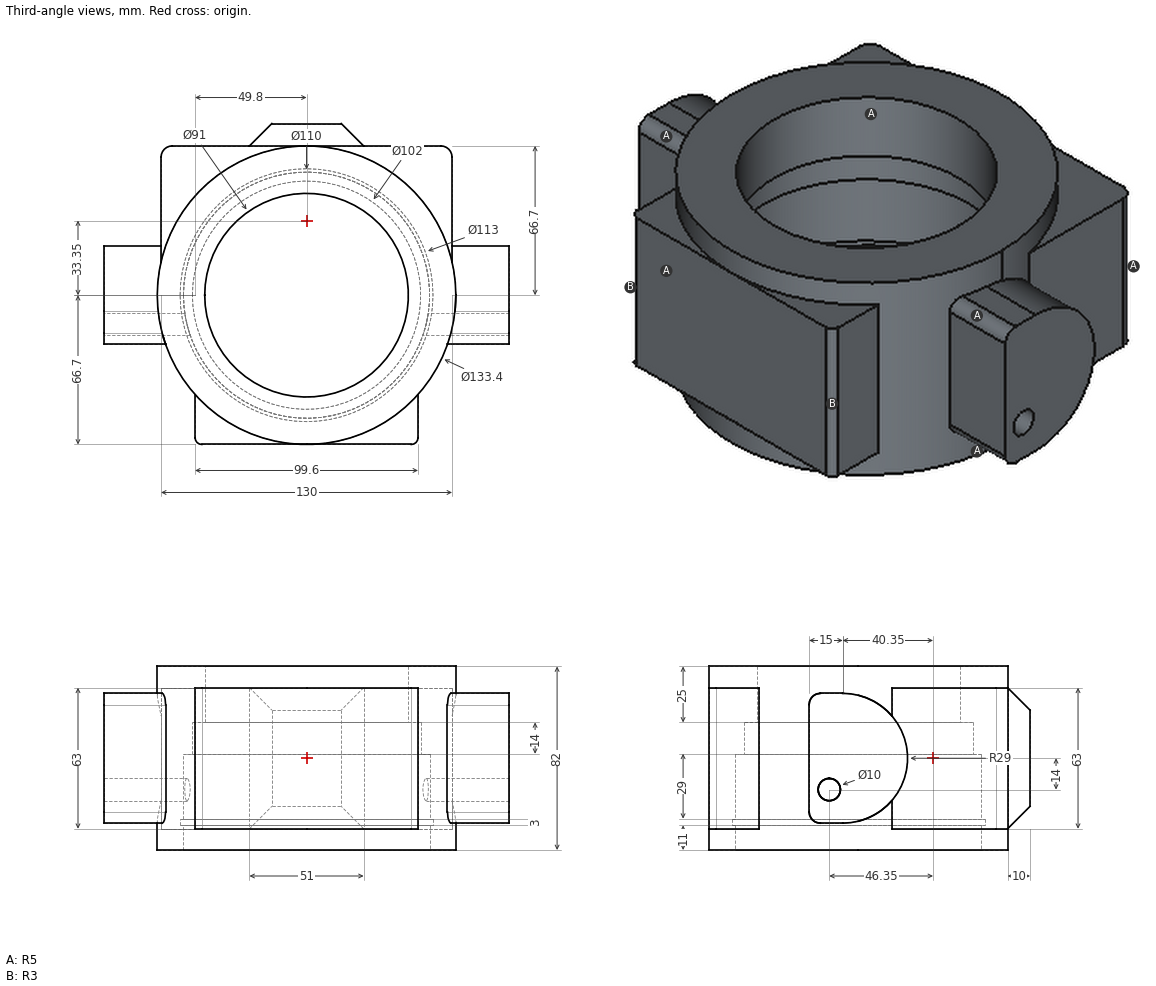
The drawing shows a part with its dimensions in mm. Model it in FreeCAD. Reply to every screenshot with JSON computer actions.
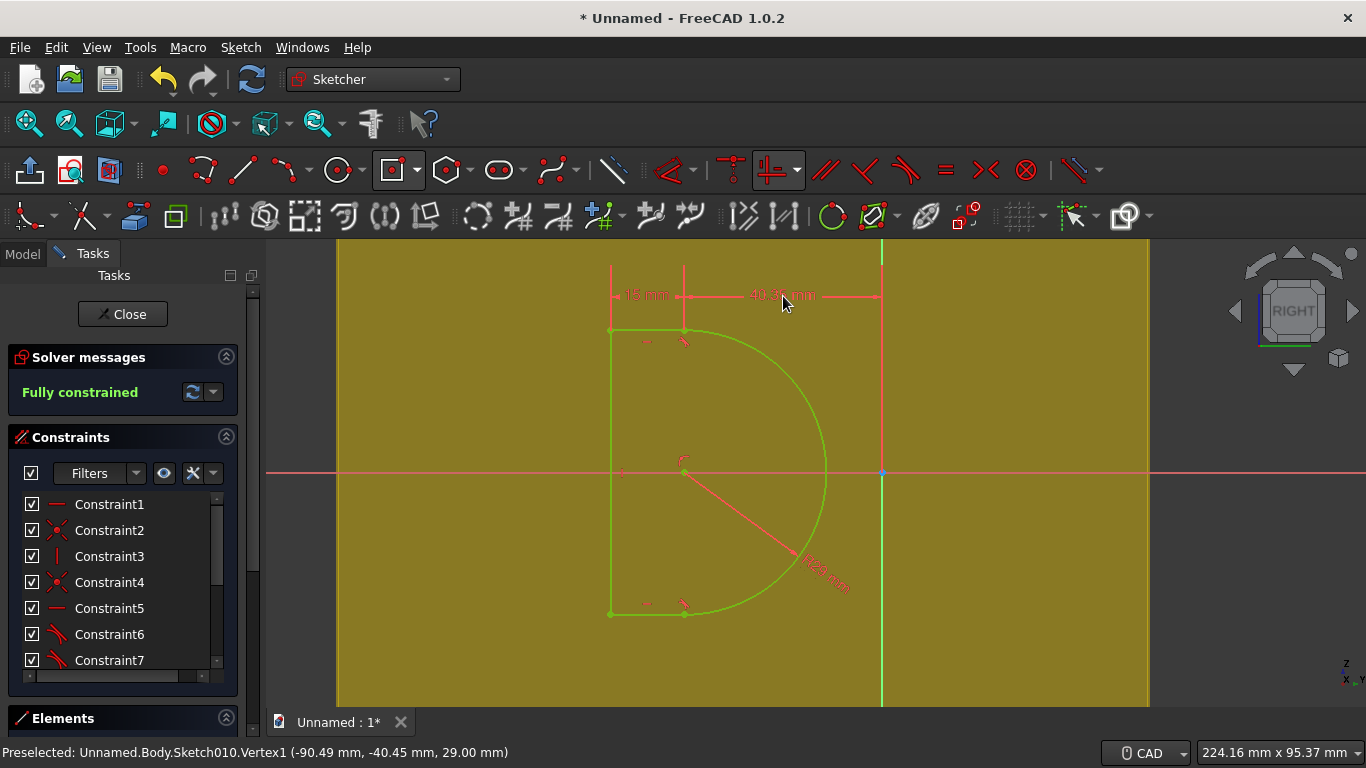
{"action": "left_click", "coordinate": [123, 314]}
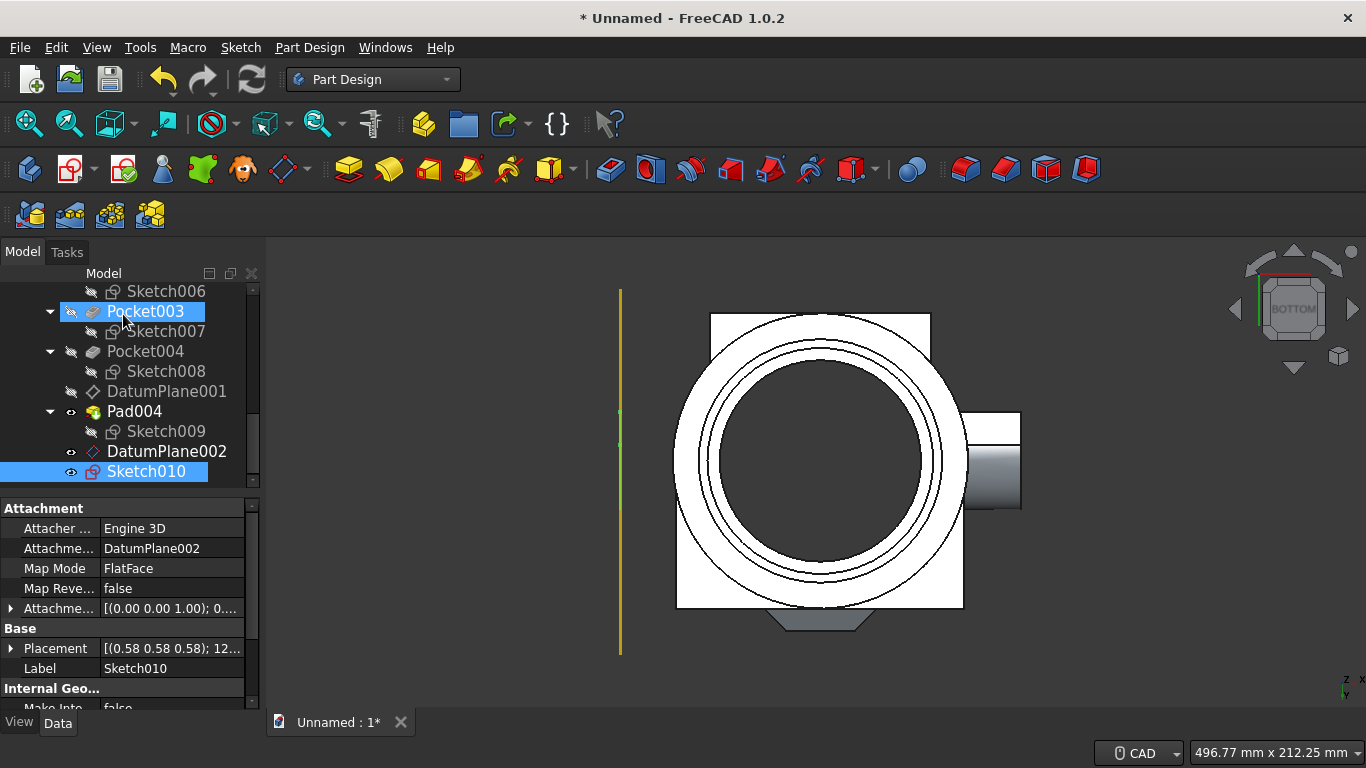
{"action": "left_click", "coordinate": [350, 170]}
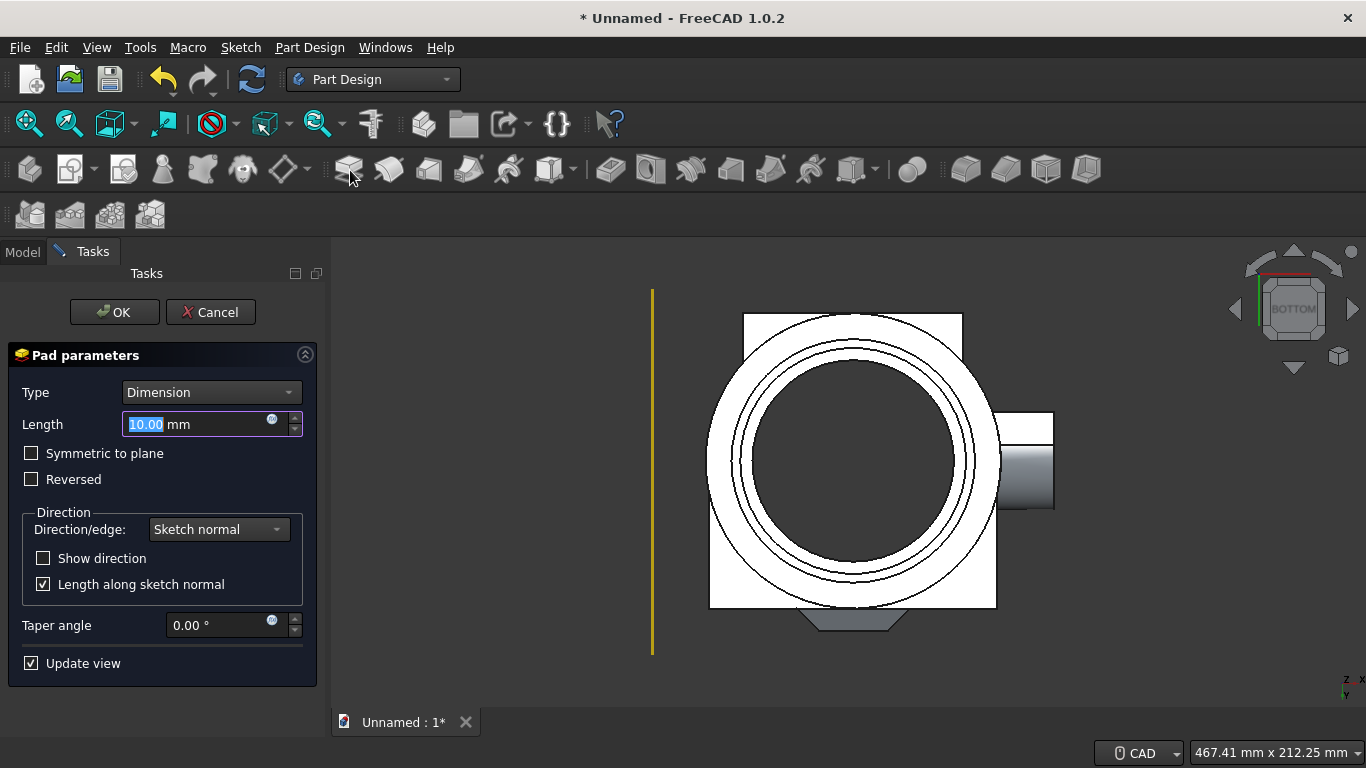
{"action": "left_click", "coordinate": [212, 392]}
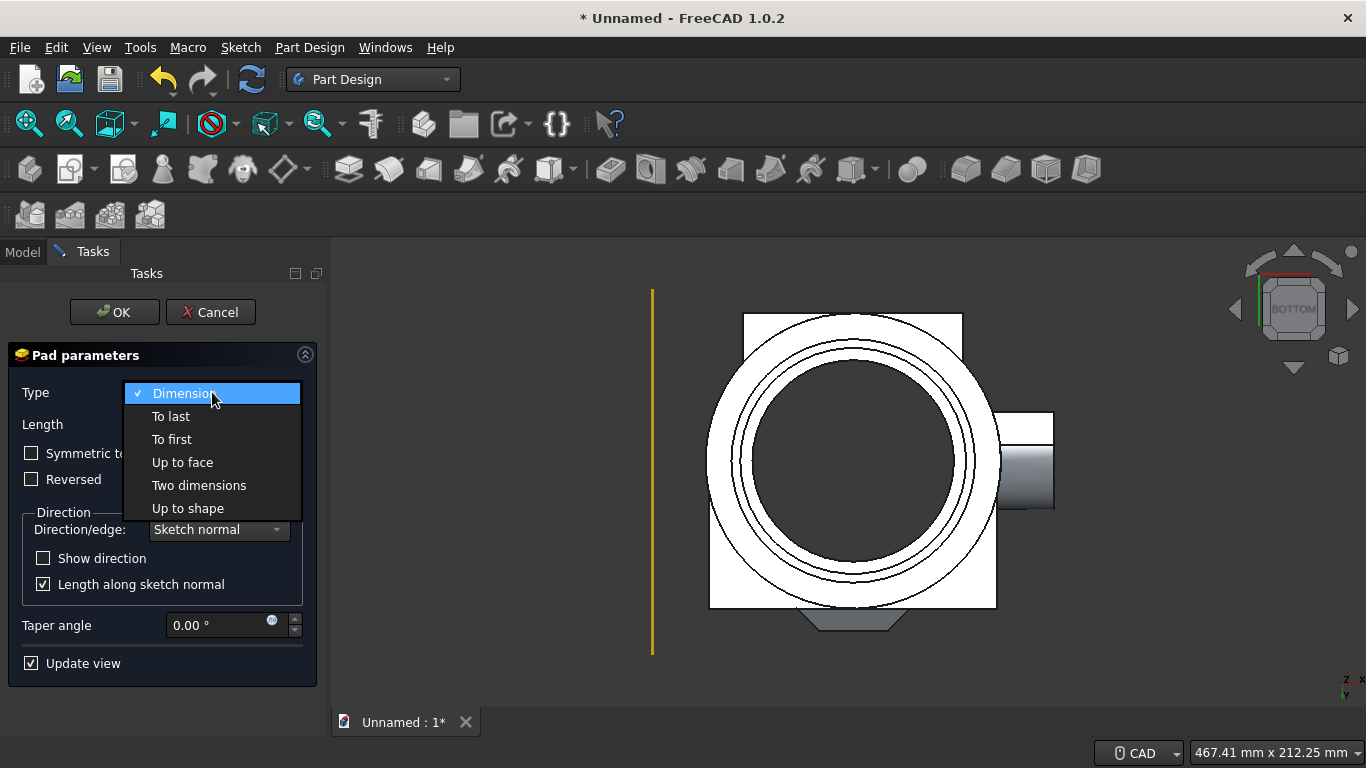
{"action": "left_click", "coordinate": [212, 440]}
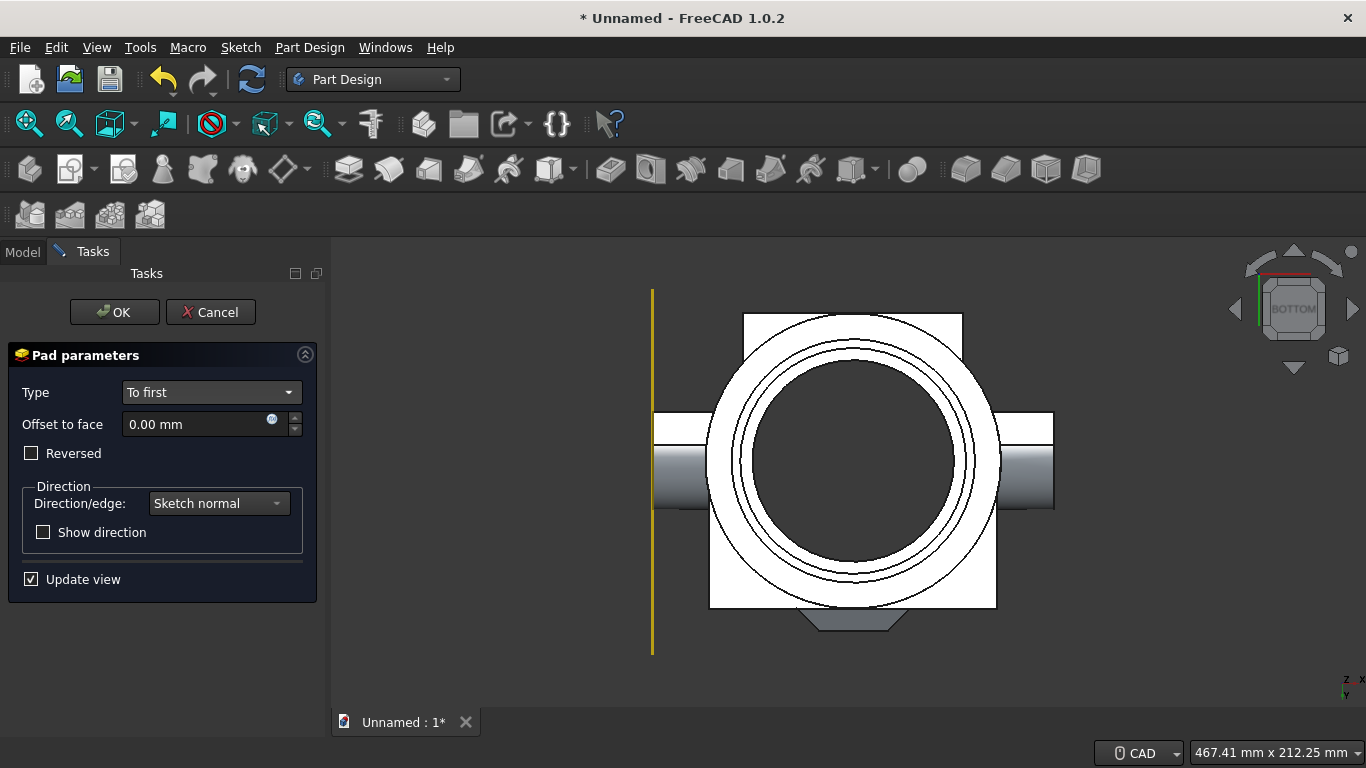
{"action": "left_click", "coordinate": [115, 312]}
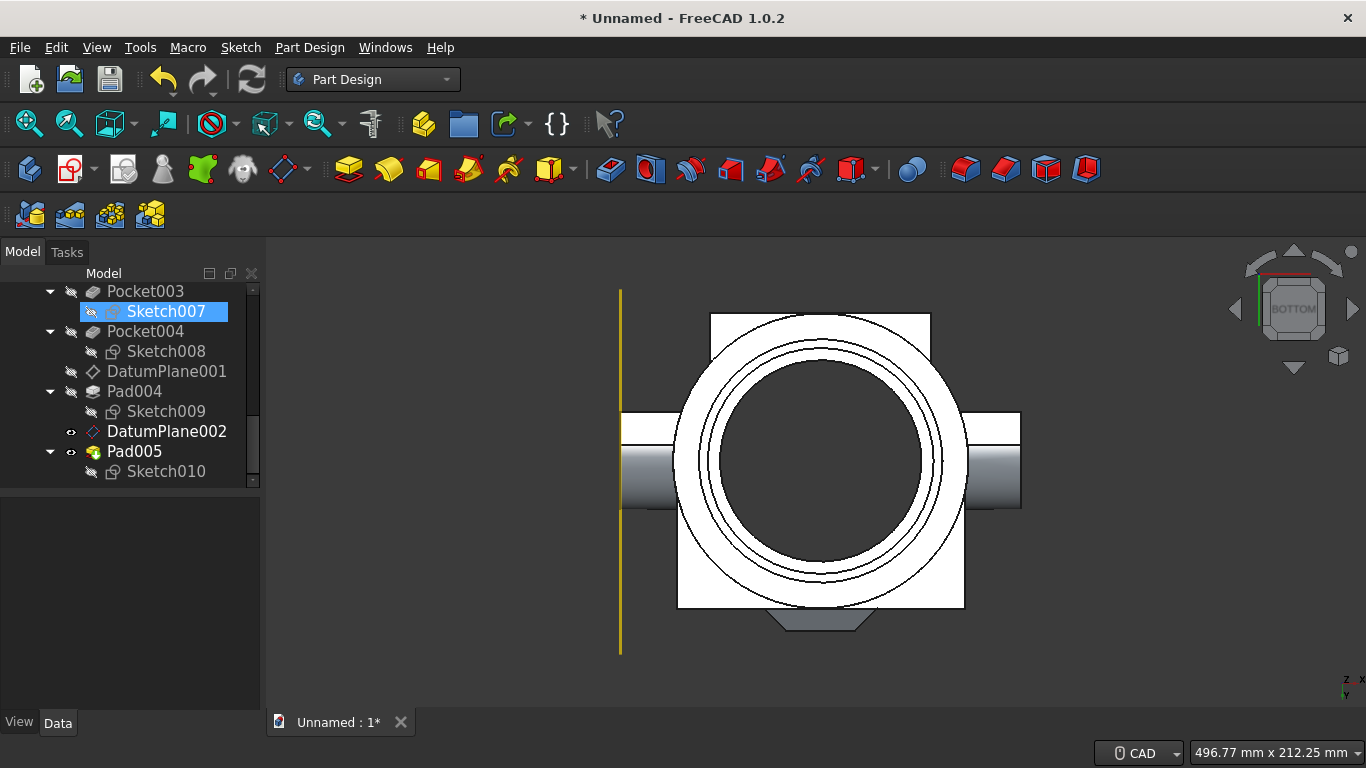
{"action": "left_click", "coordinate": [116, 432]}
{"action": "key", "text": "space"}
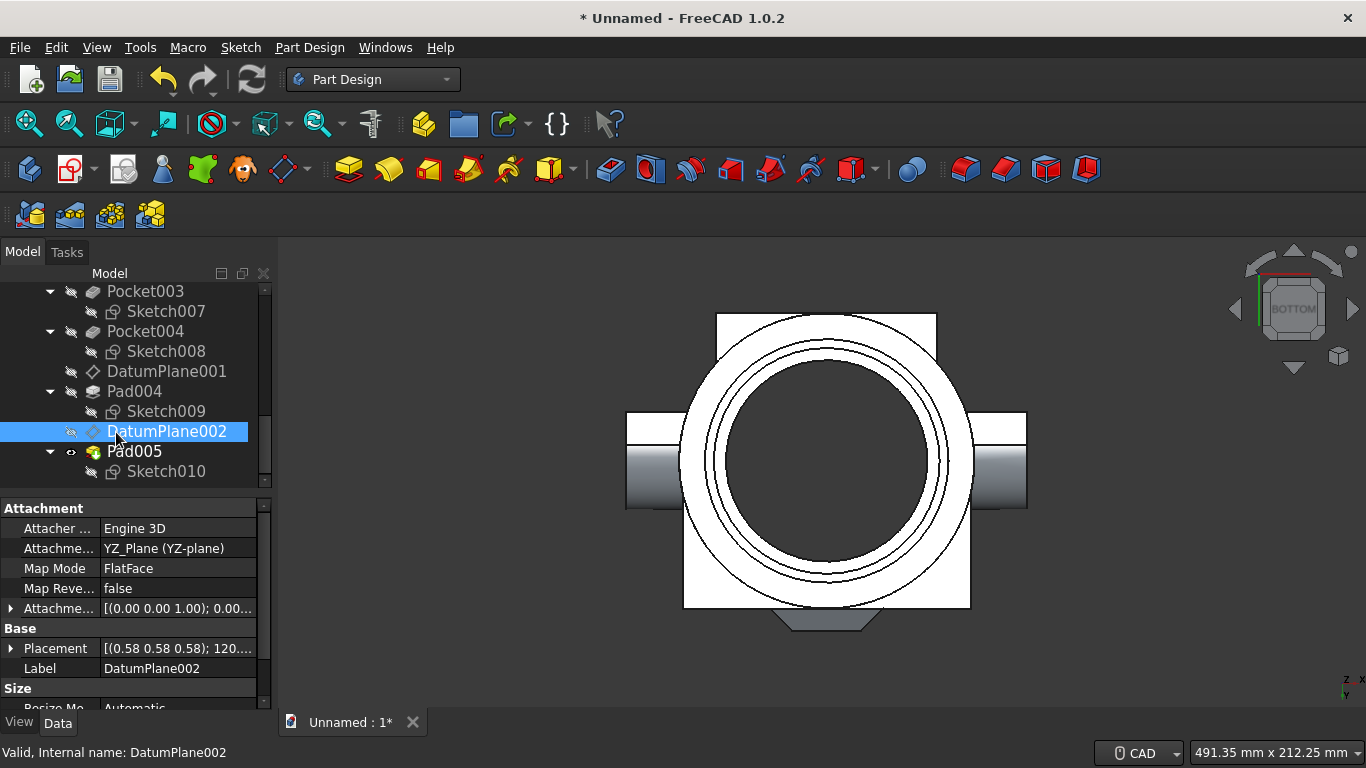
{"action": "key", "text": "6"}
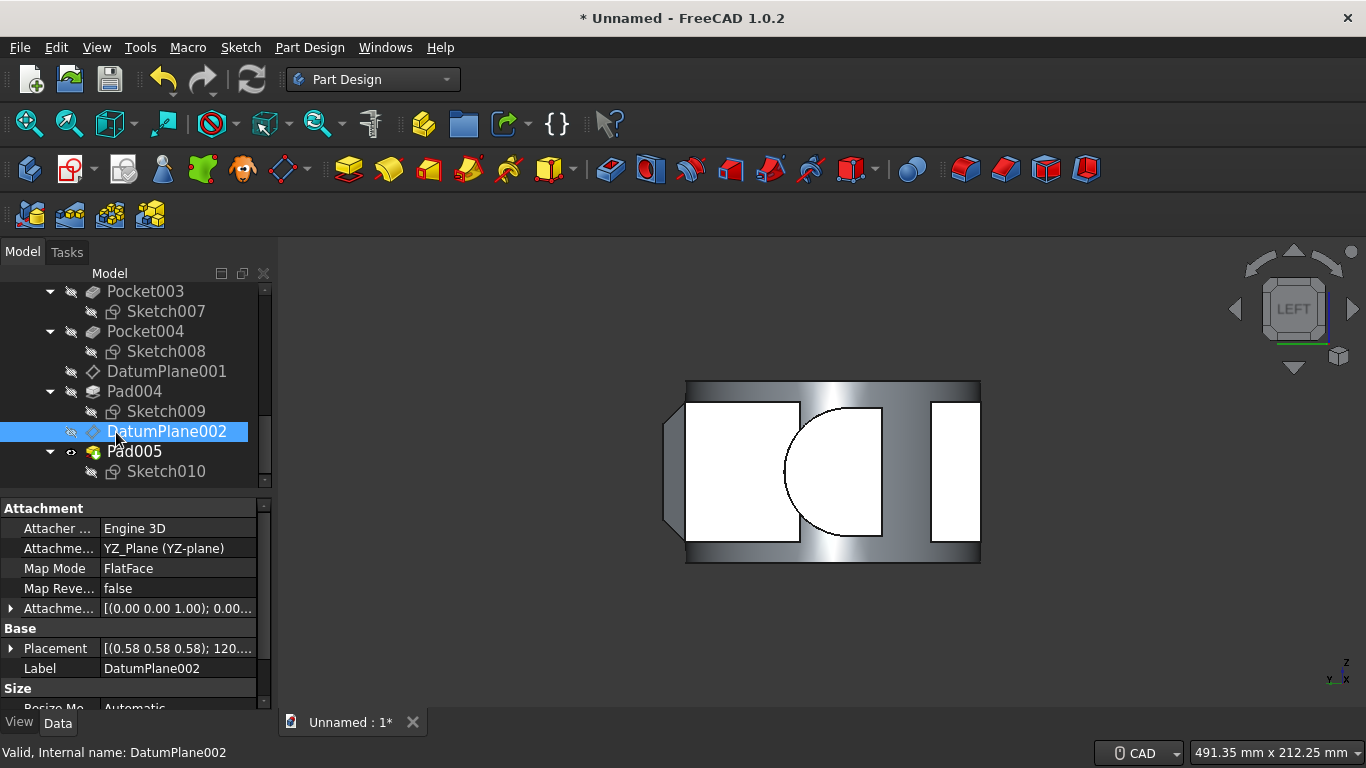
{"action": "left_click", "coordinate": [30, 124]}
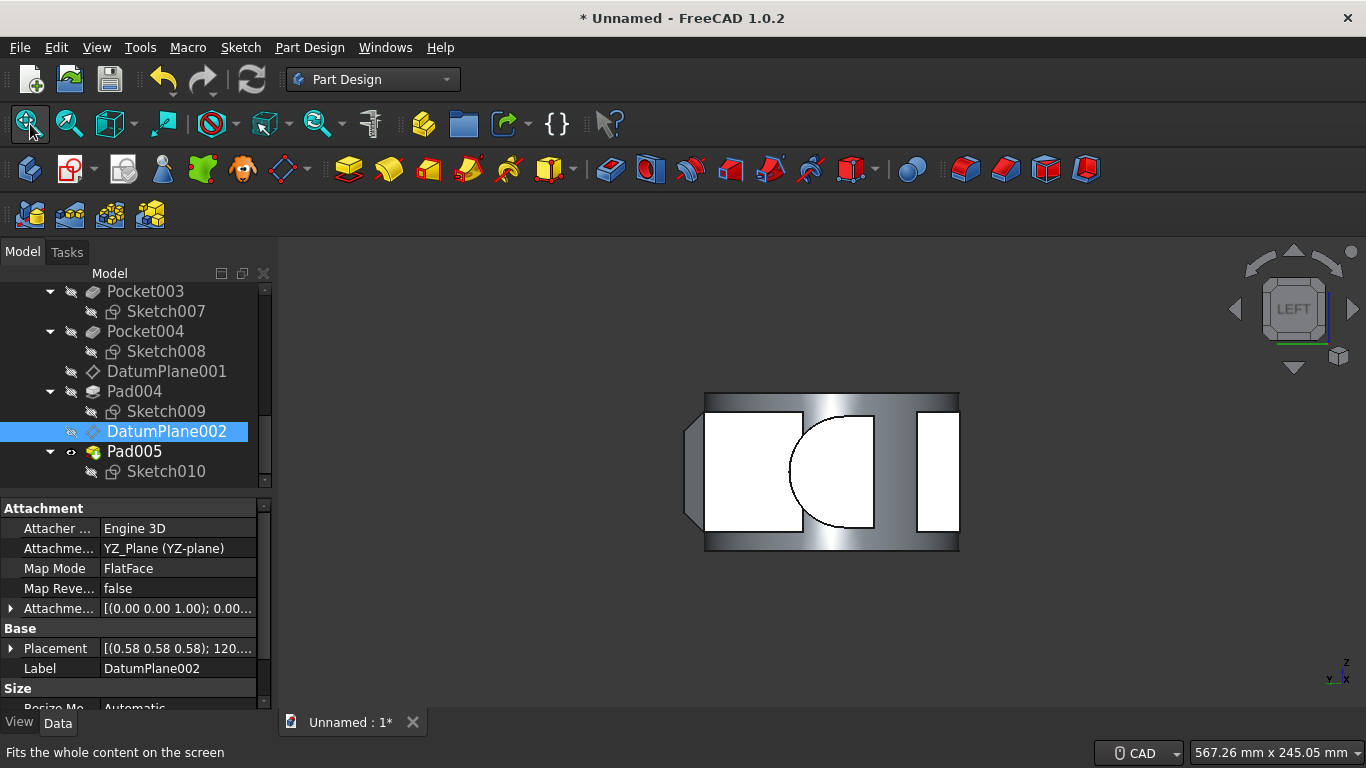
{"action": "left_click", "coordinate": [832, 471]}